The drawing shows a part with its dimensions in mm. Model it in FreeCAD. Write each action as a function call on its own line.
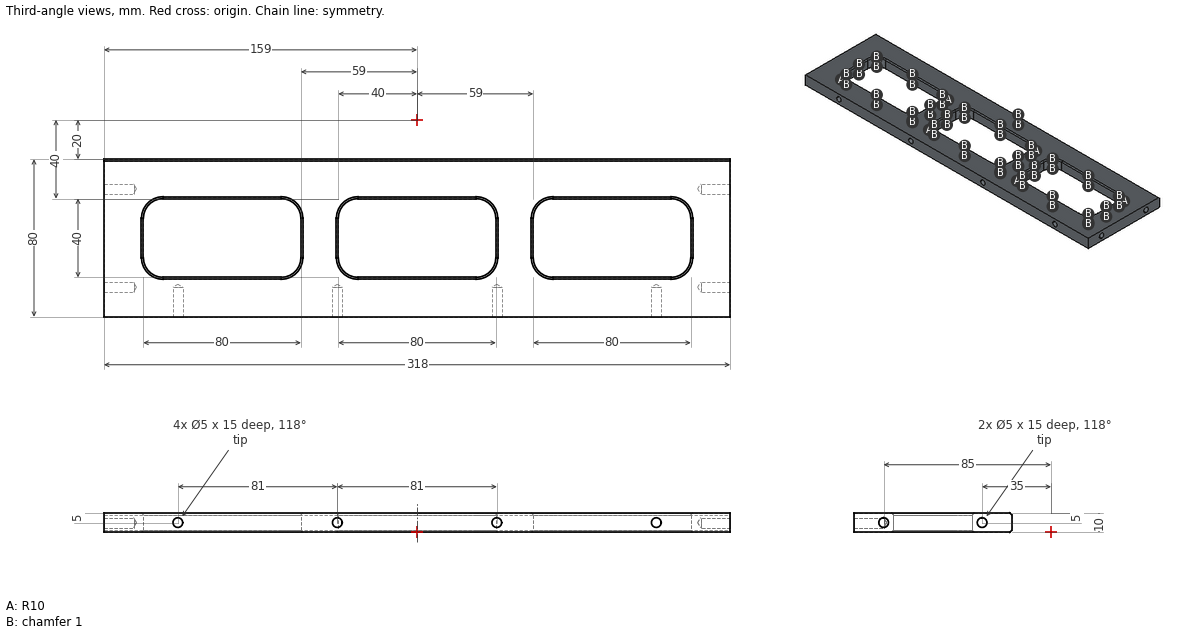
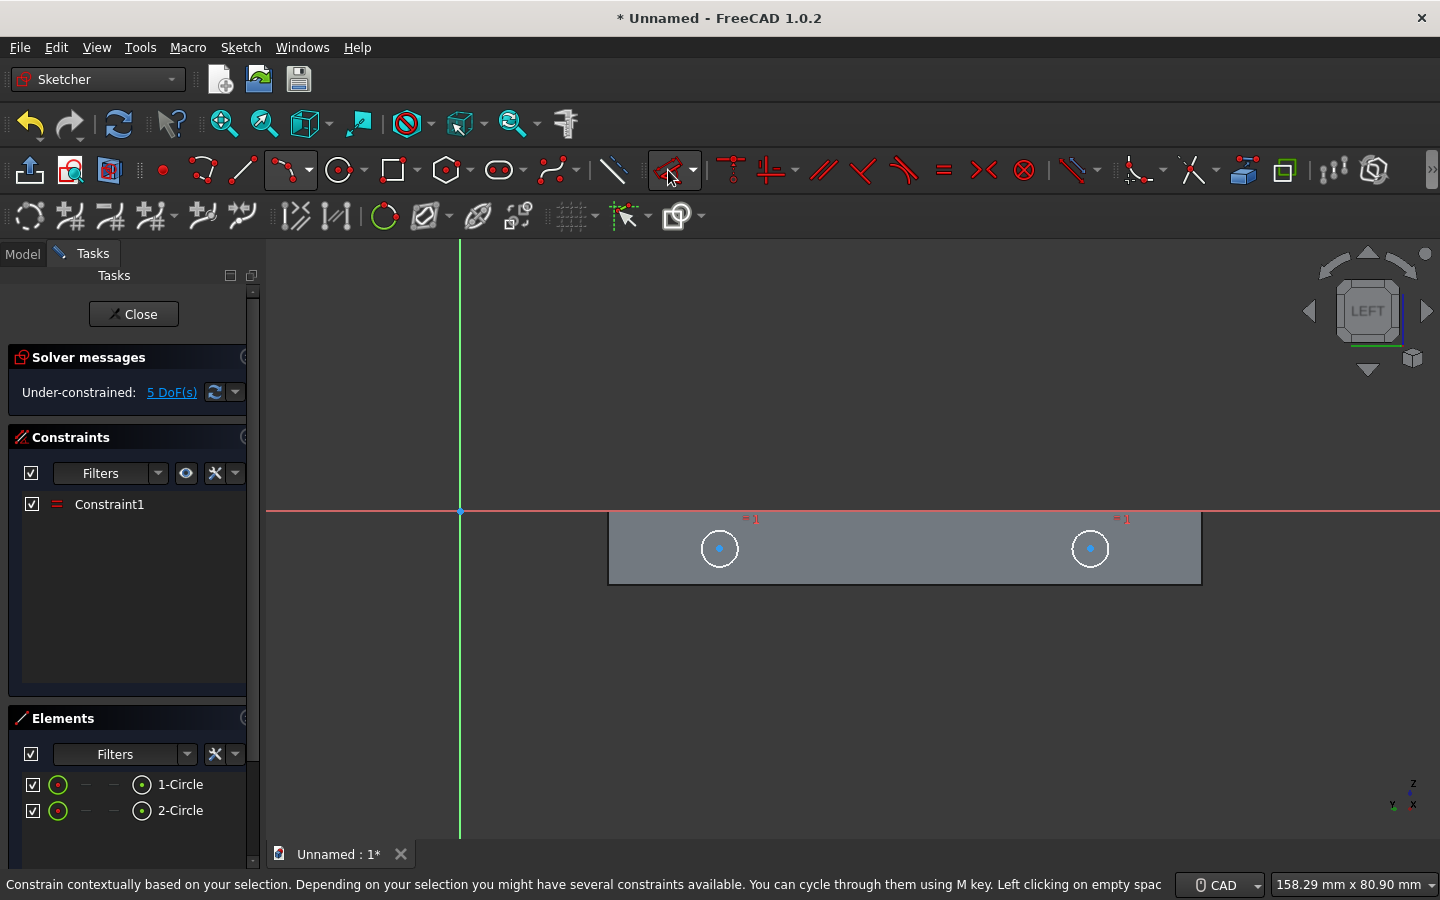
click(732, 536)
click(767, 534)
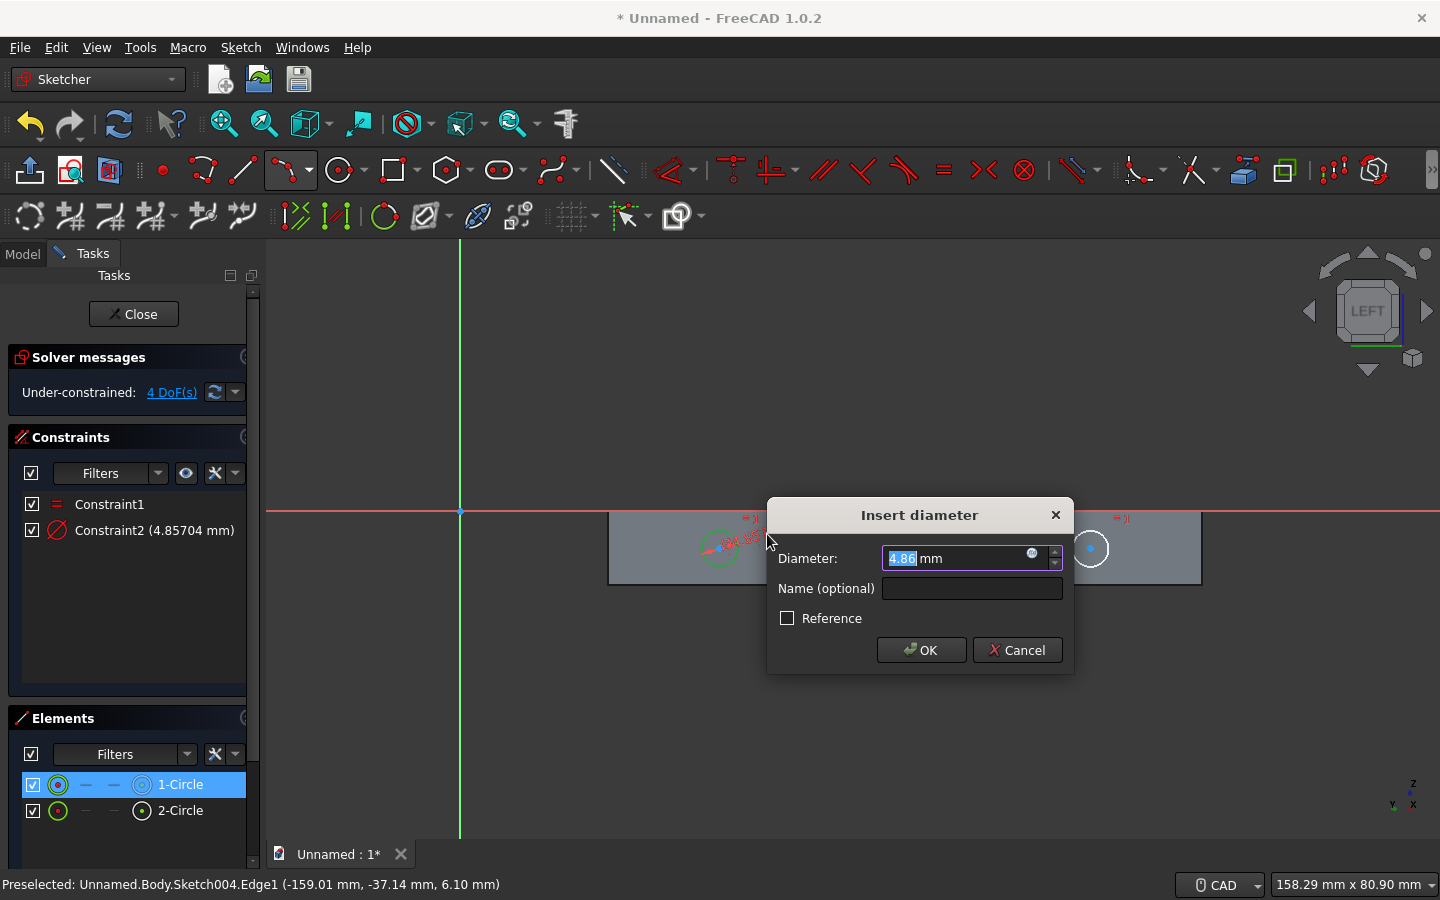
text(5)
key(Return)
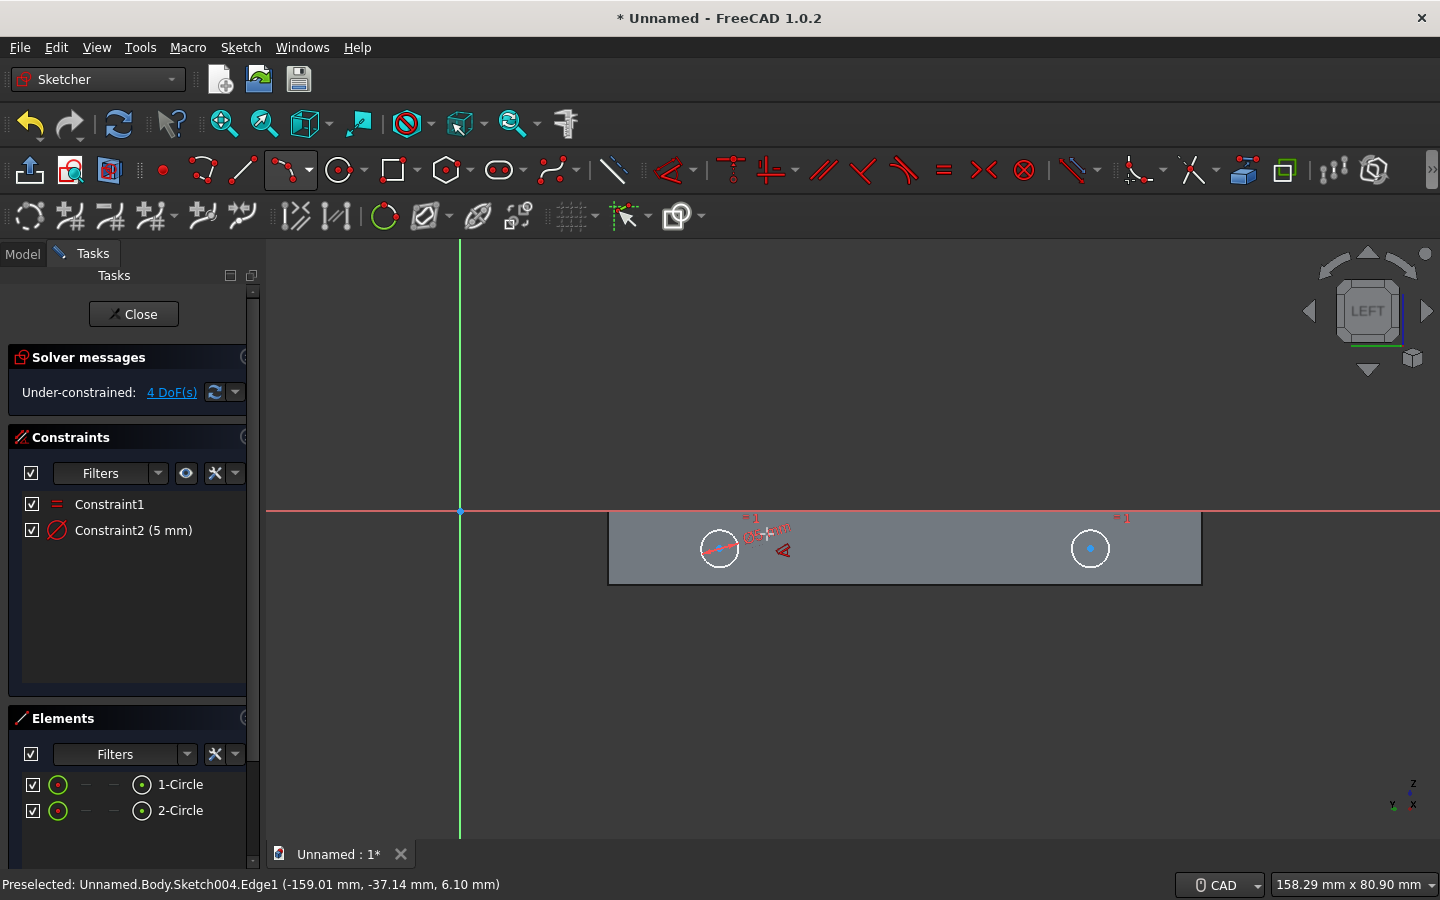
click(720, 549)
click(426, 530)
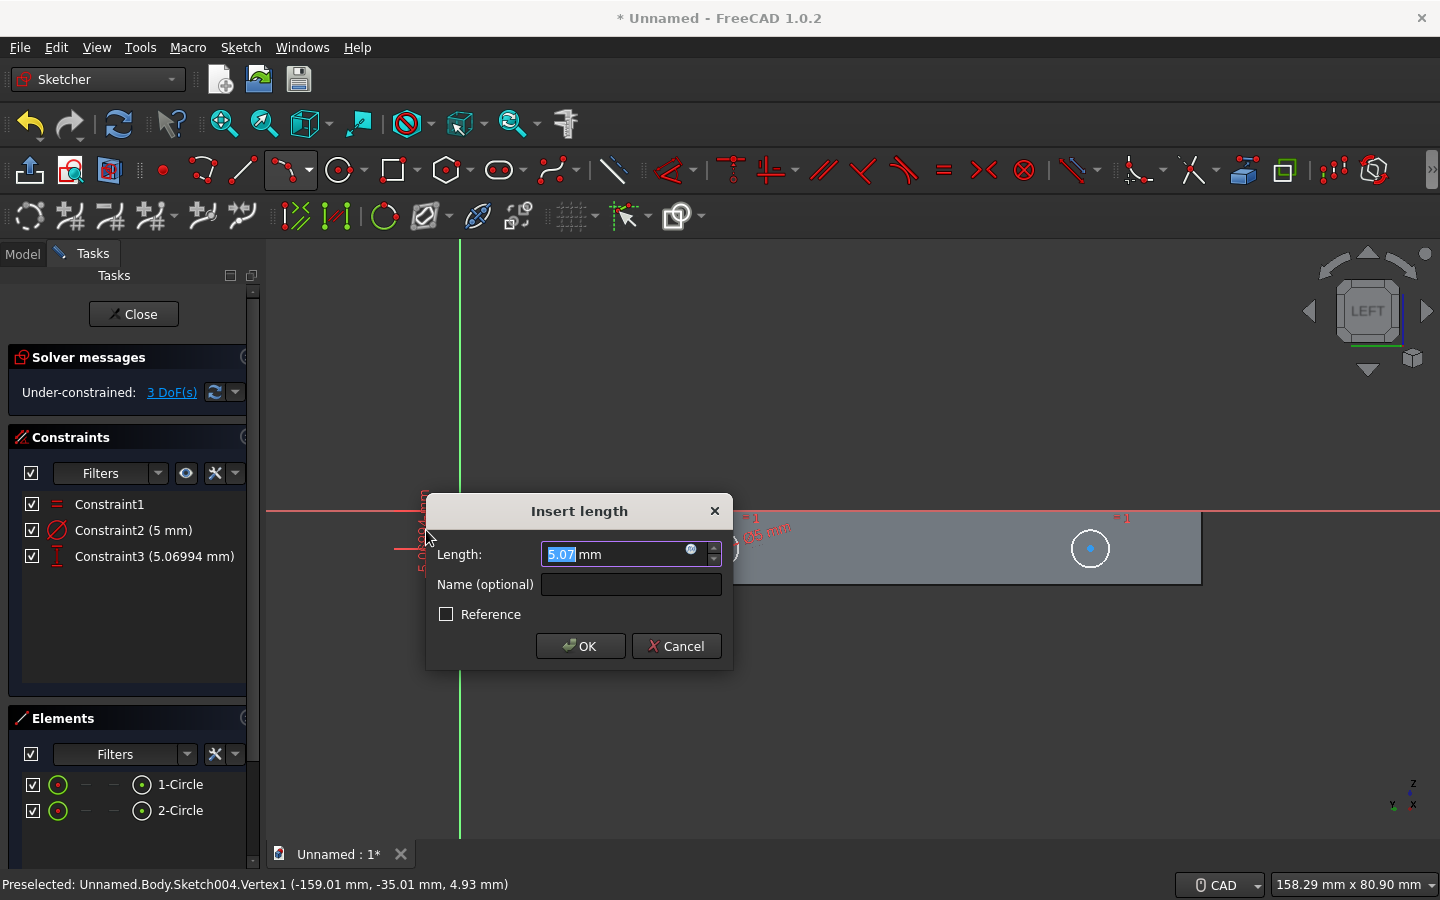
text(5)
key(Return)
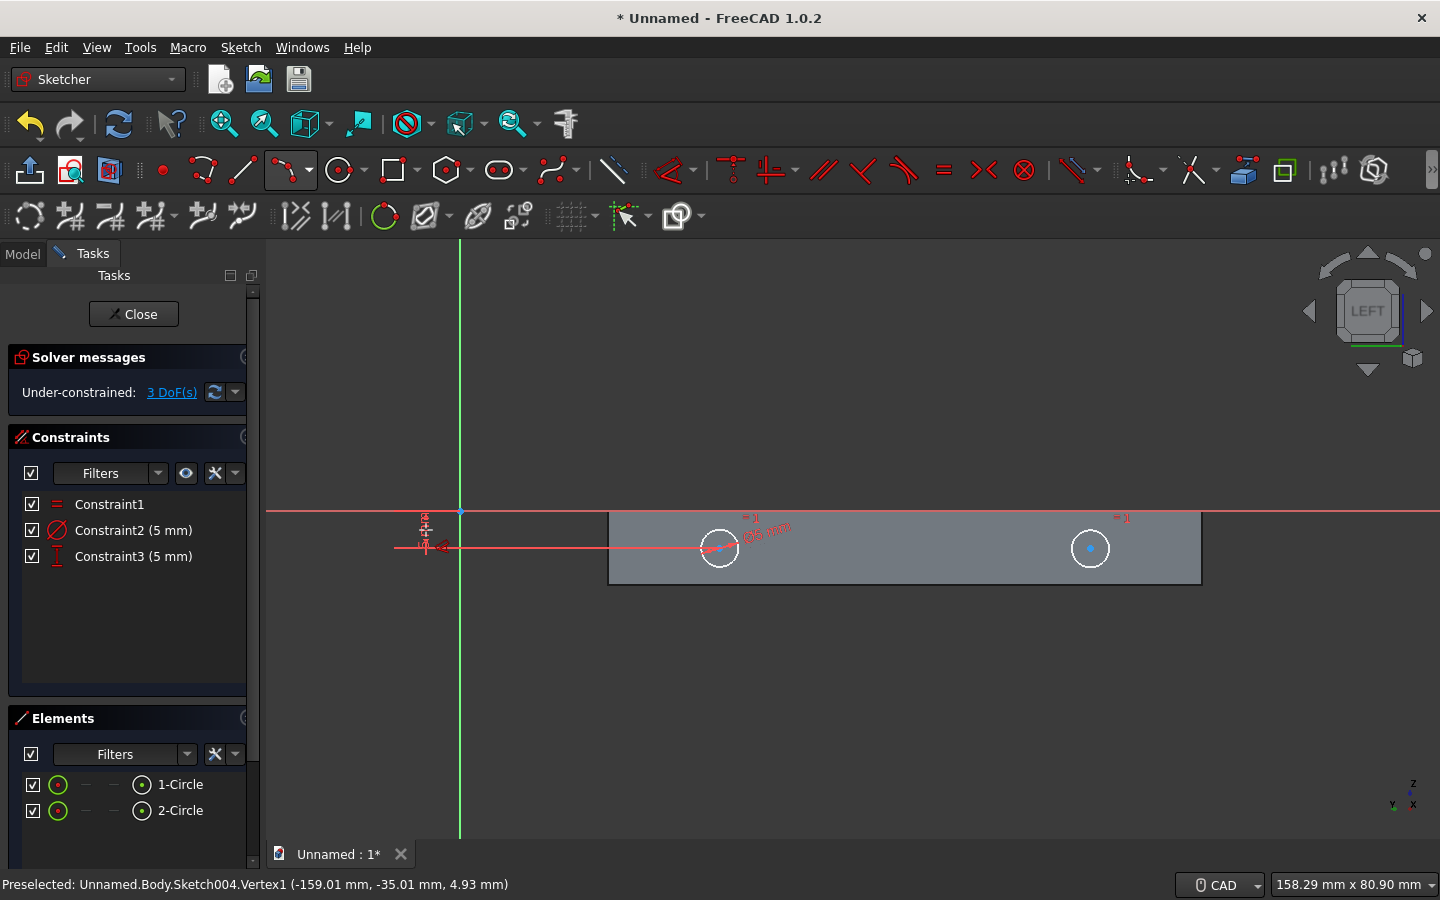
click(1090, 549)
click(1124, 530)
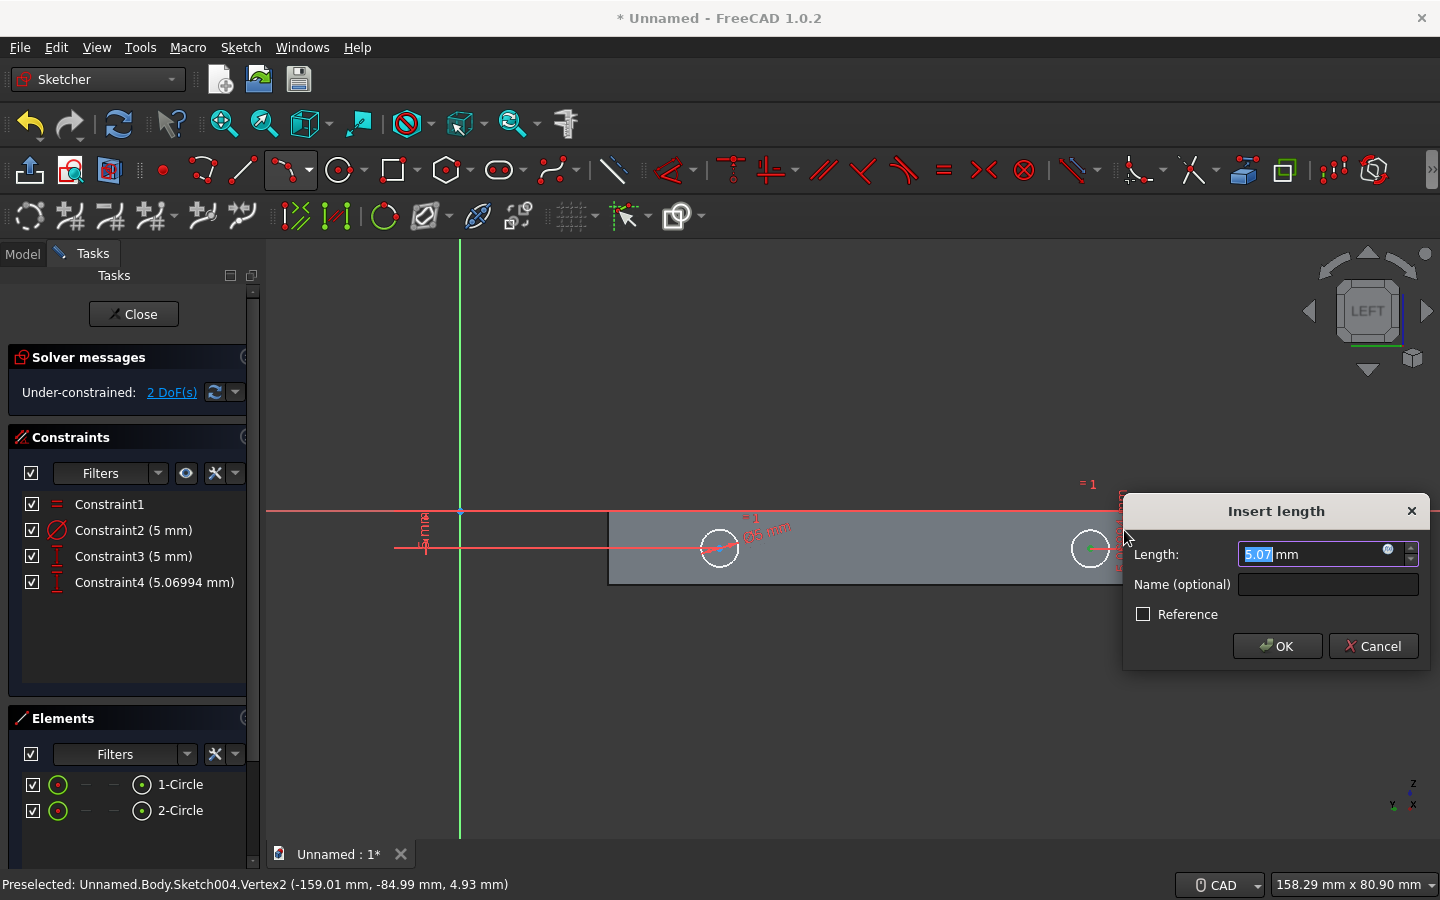
text(5)
key(Return)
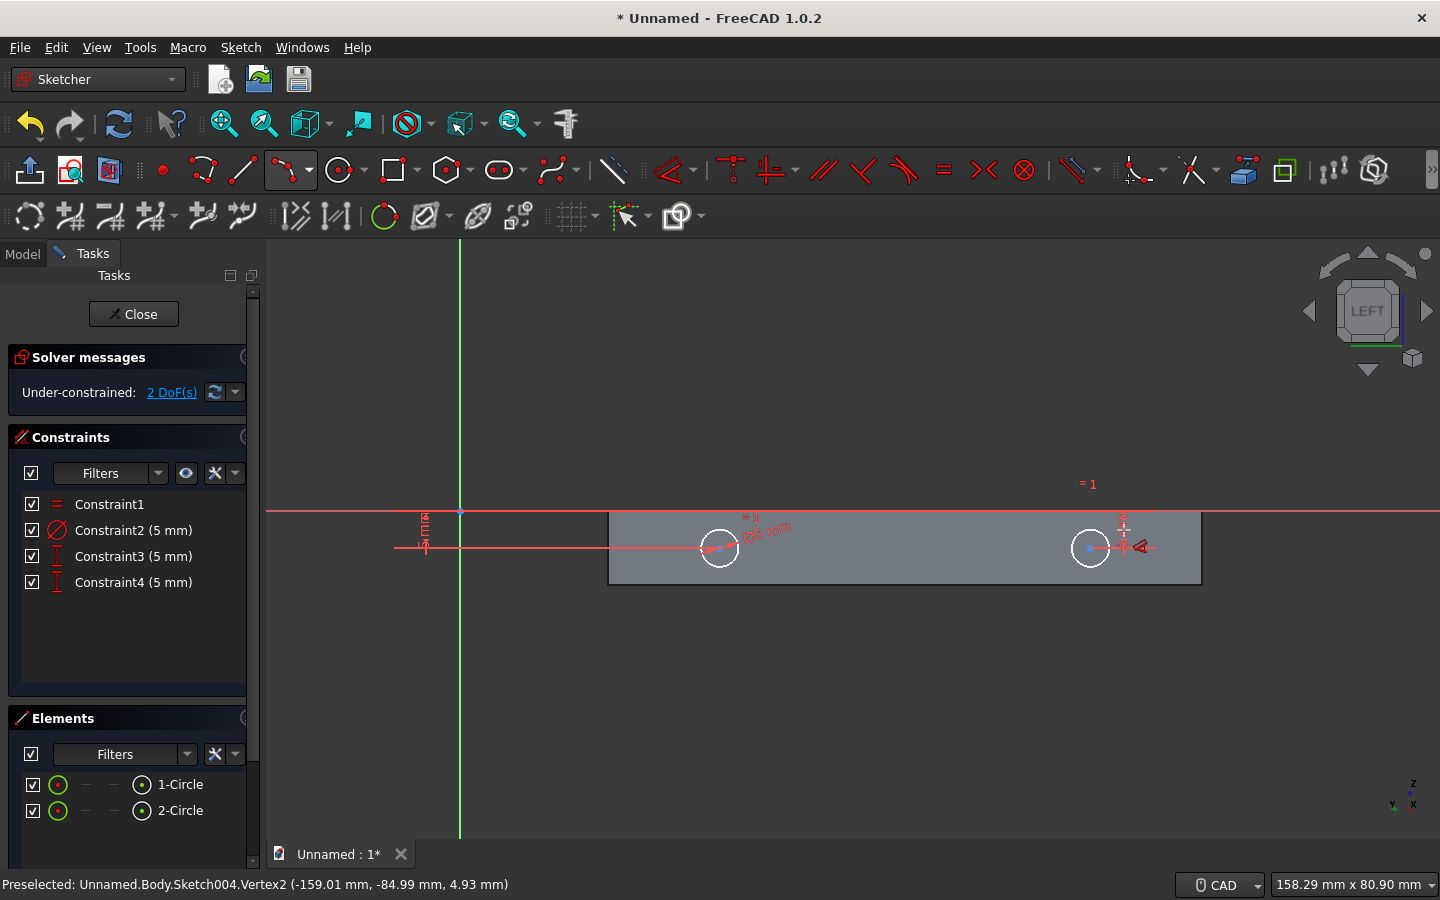
click(720, 548)
click(590, 477)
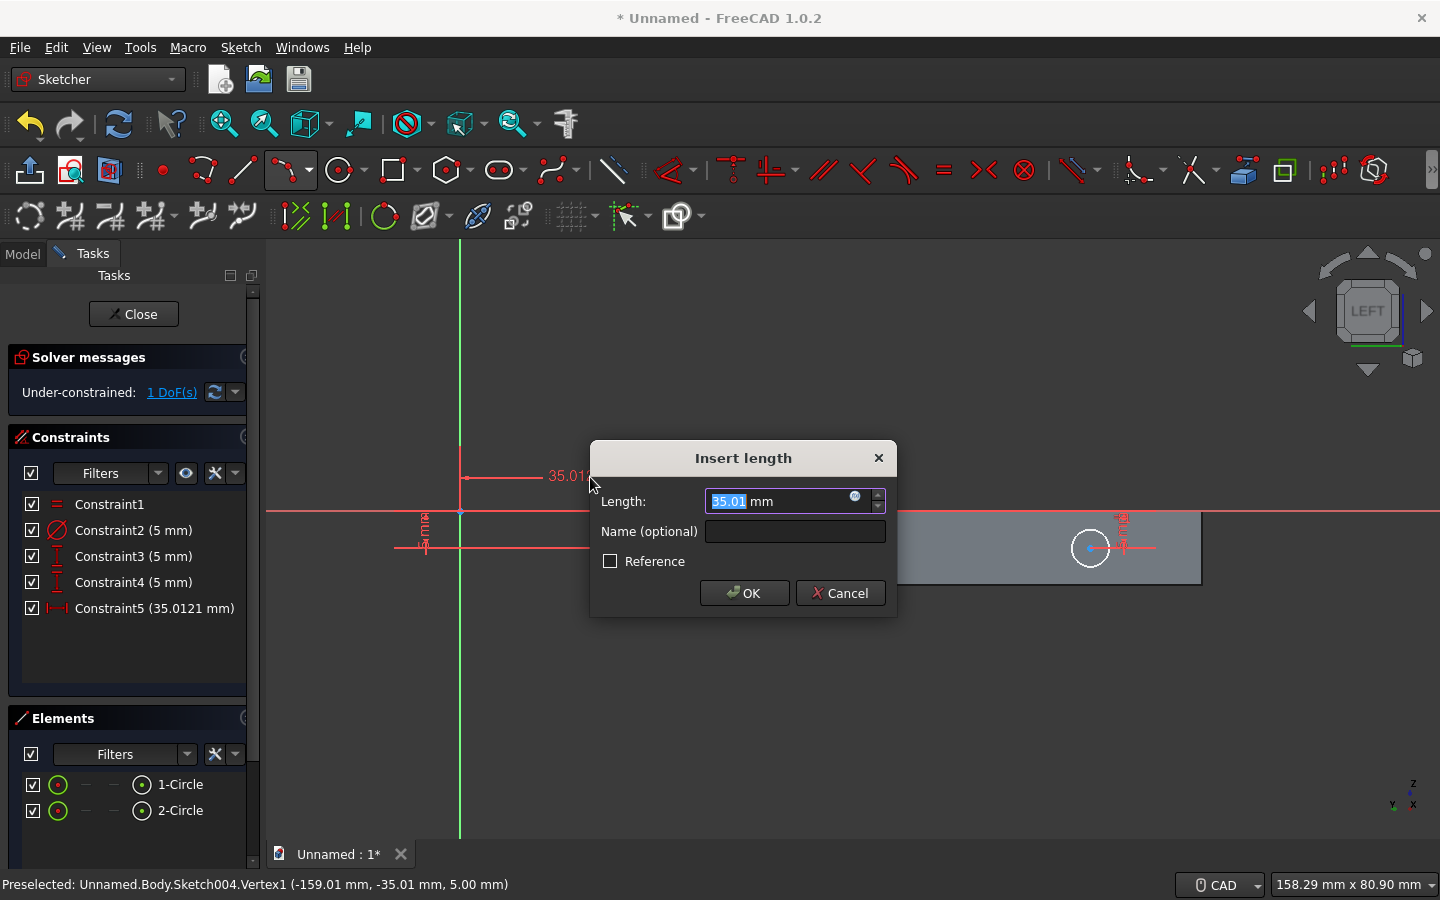
text(35)
key(Return)